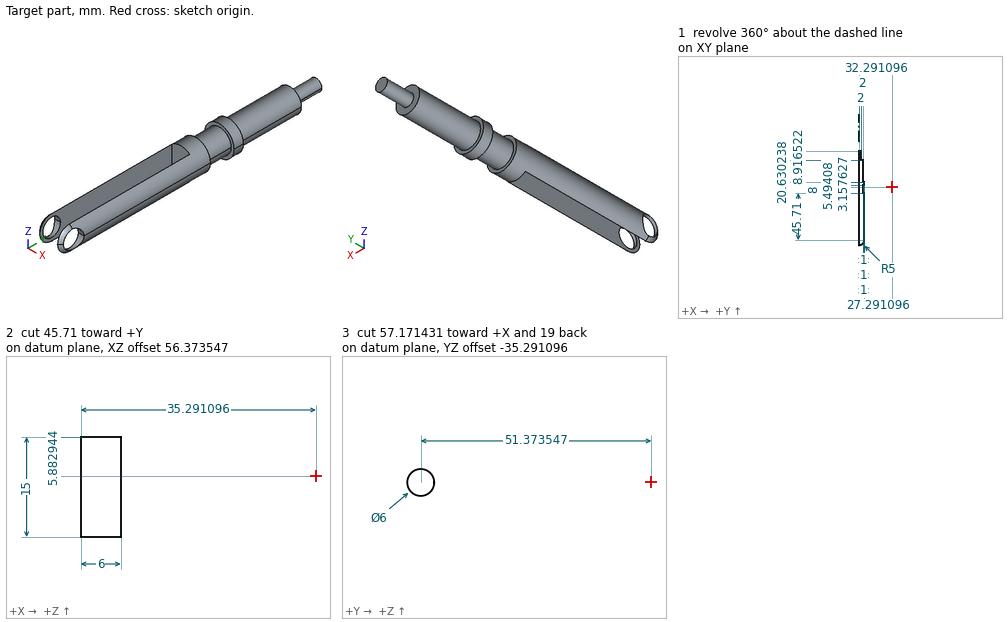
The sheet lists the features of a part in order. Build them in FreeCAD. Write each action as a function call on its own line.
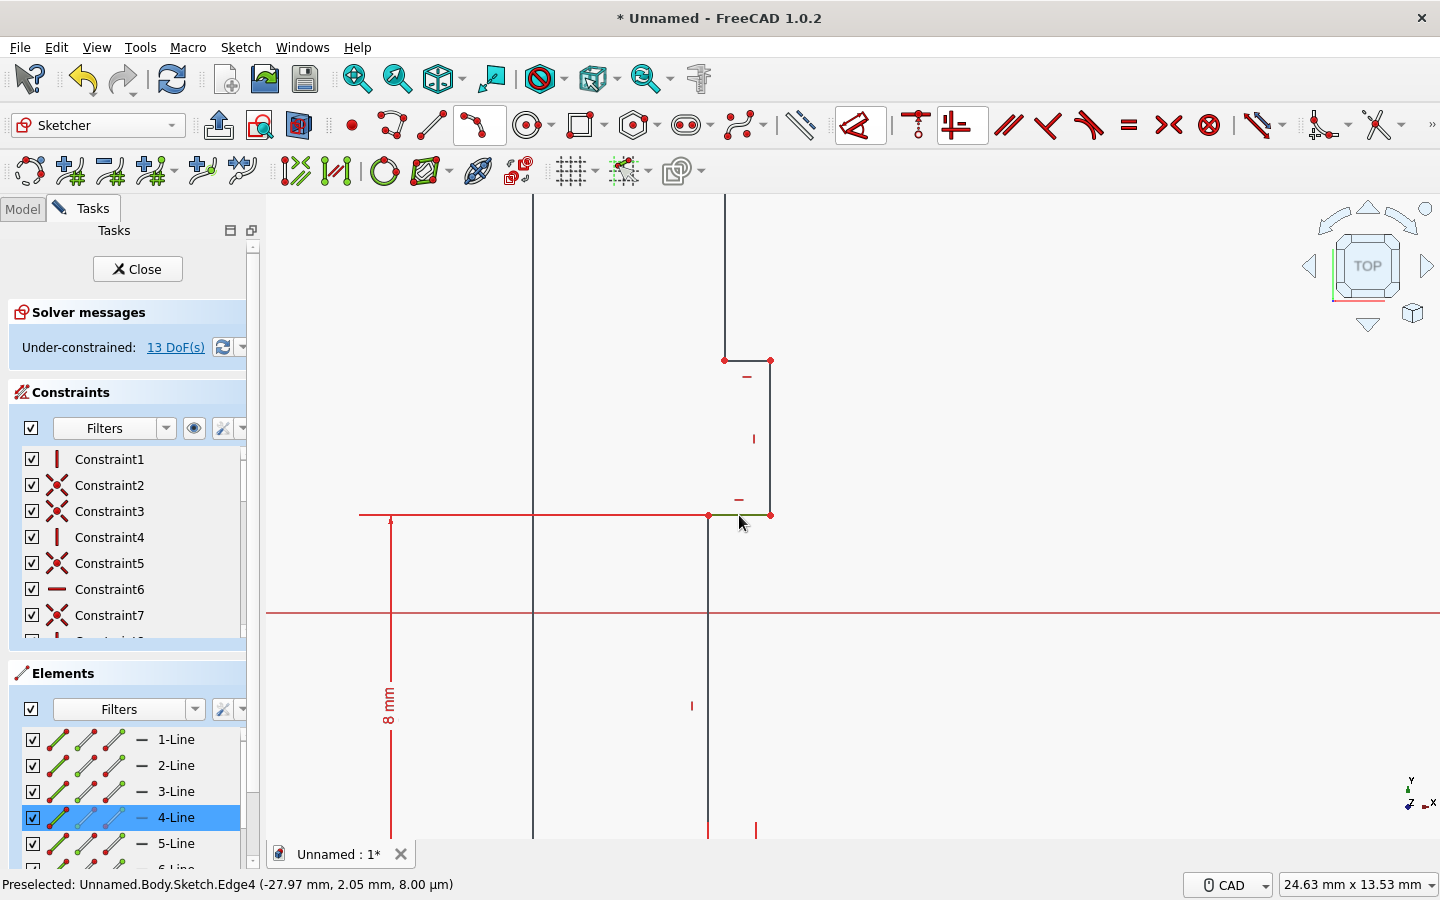
key(l)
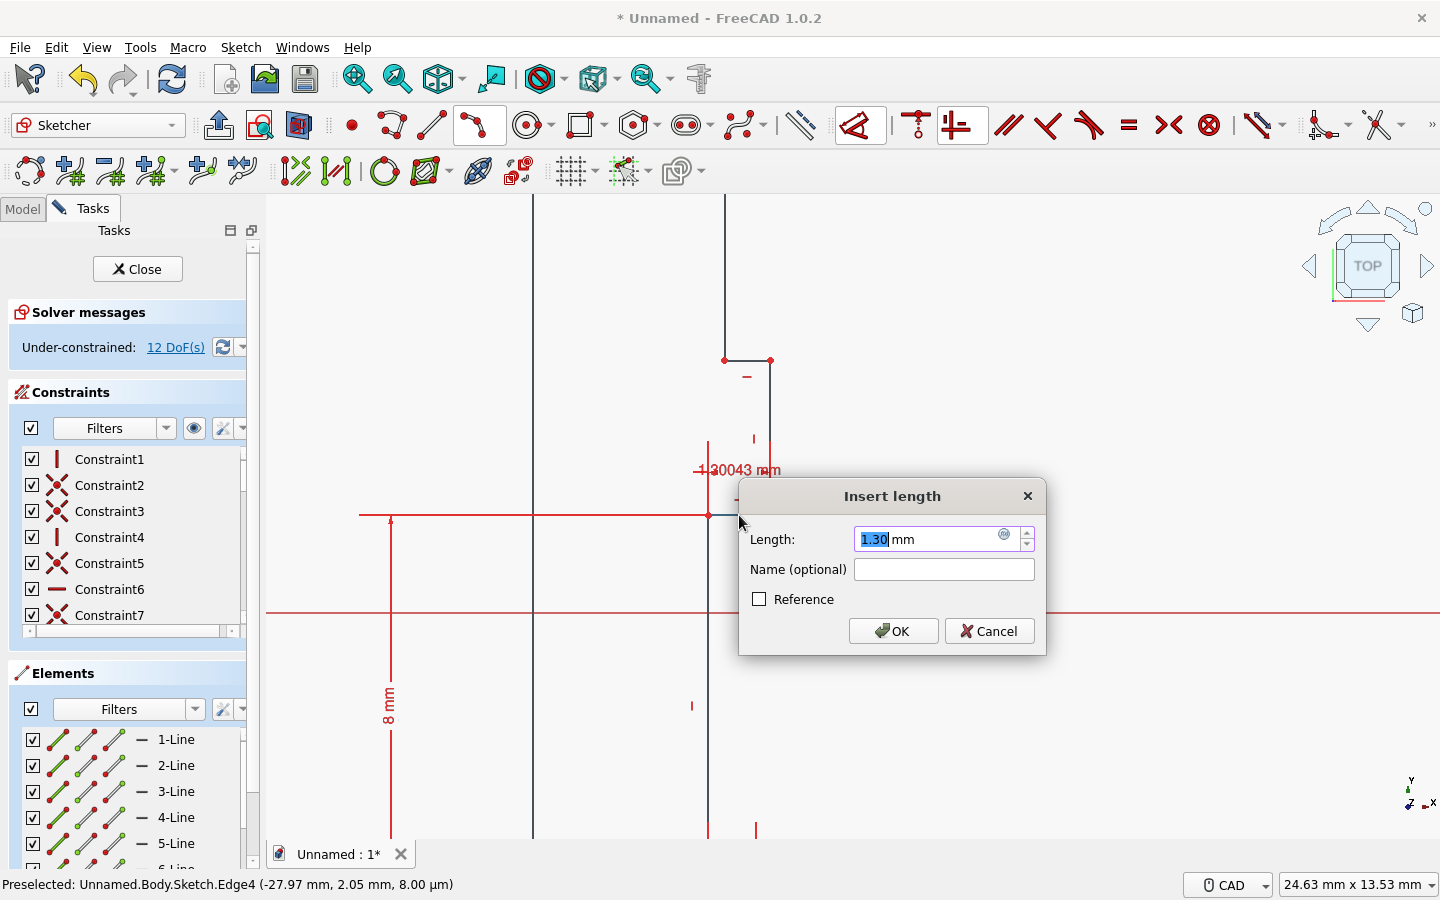
text(1)
key(Return)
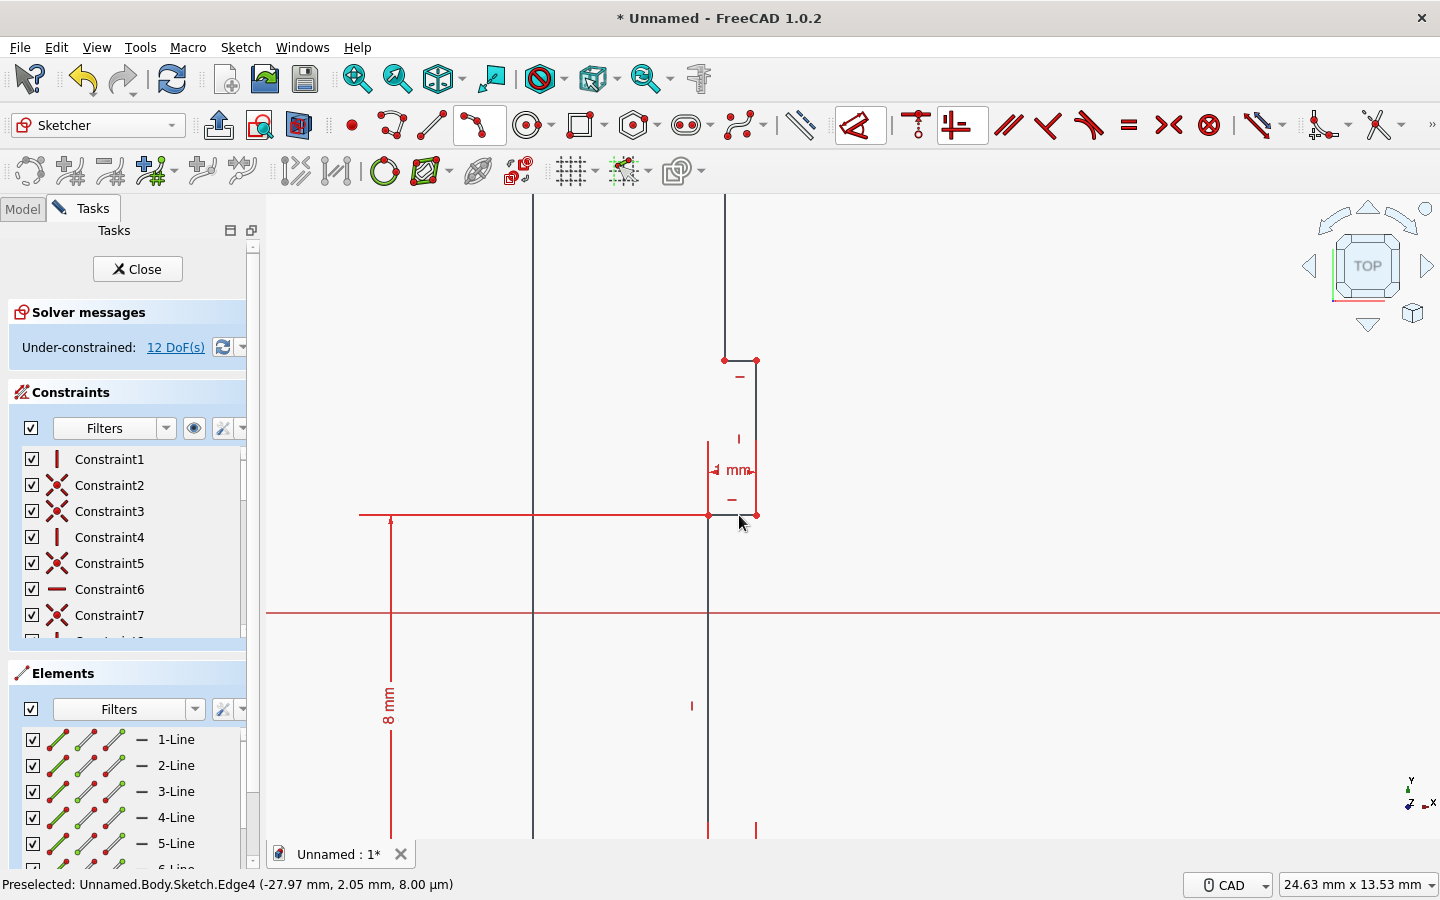
click(747, 361)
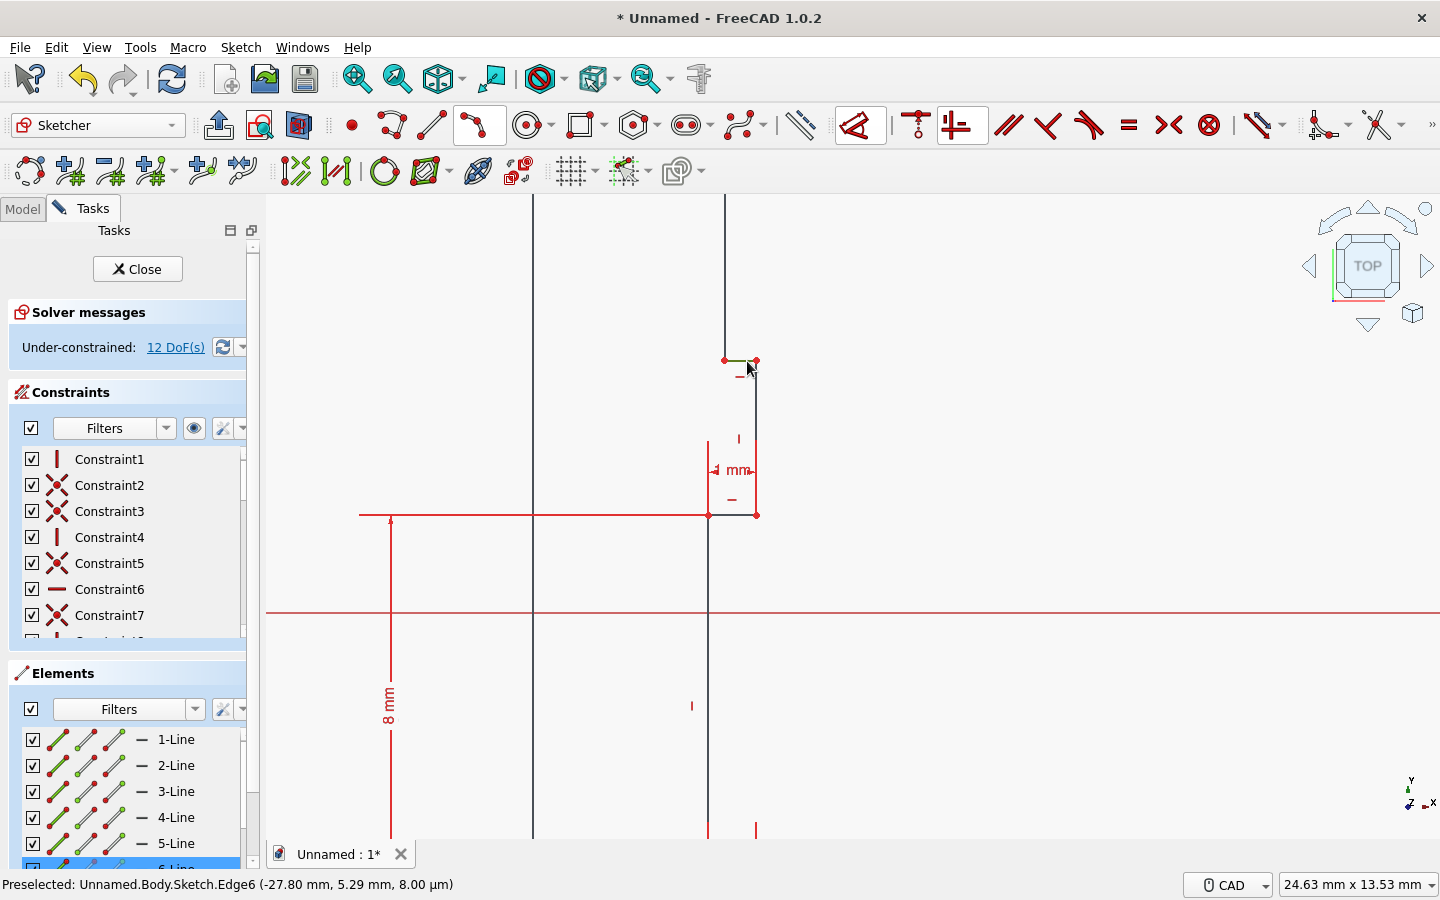
click(880, 126)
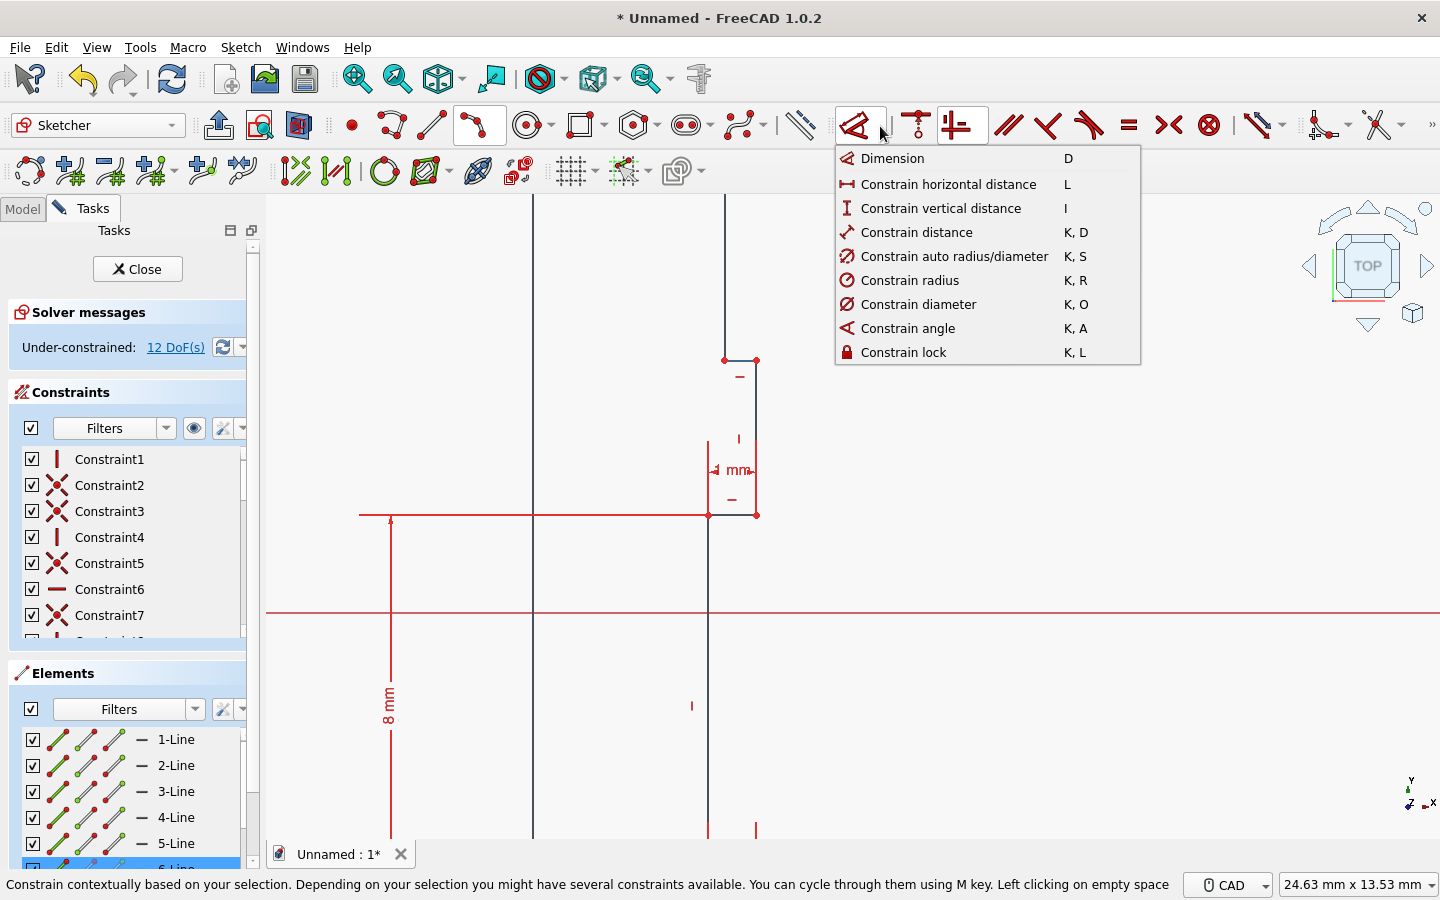
click(988, 184)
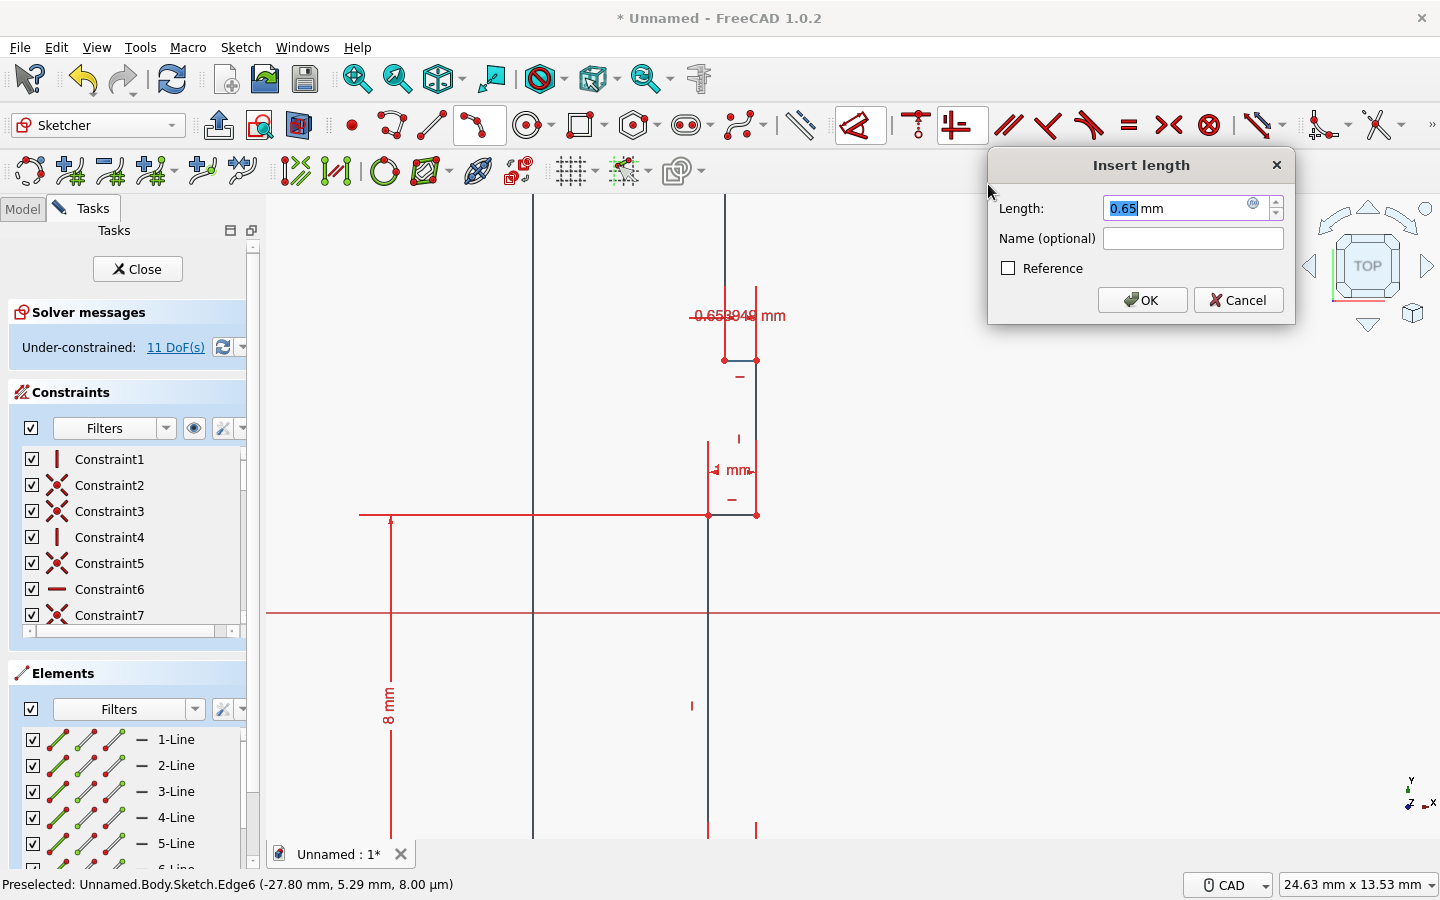
text(1)
key(Return)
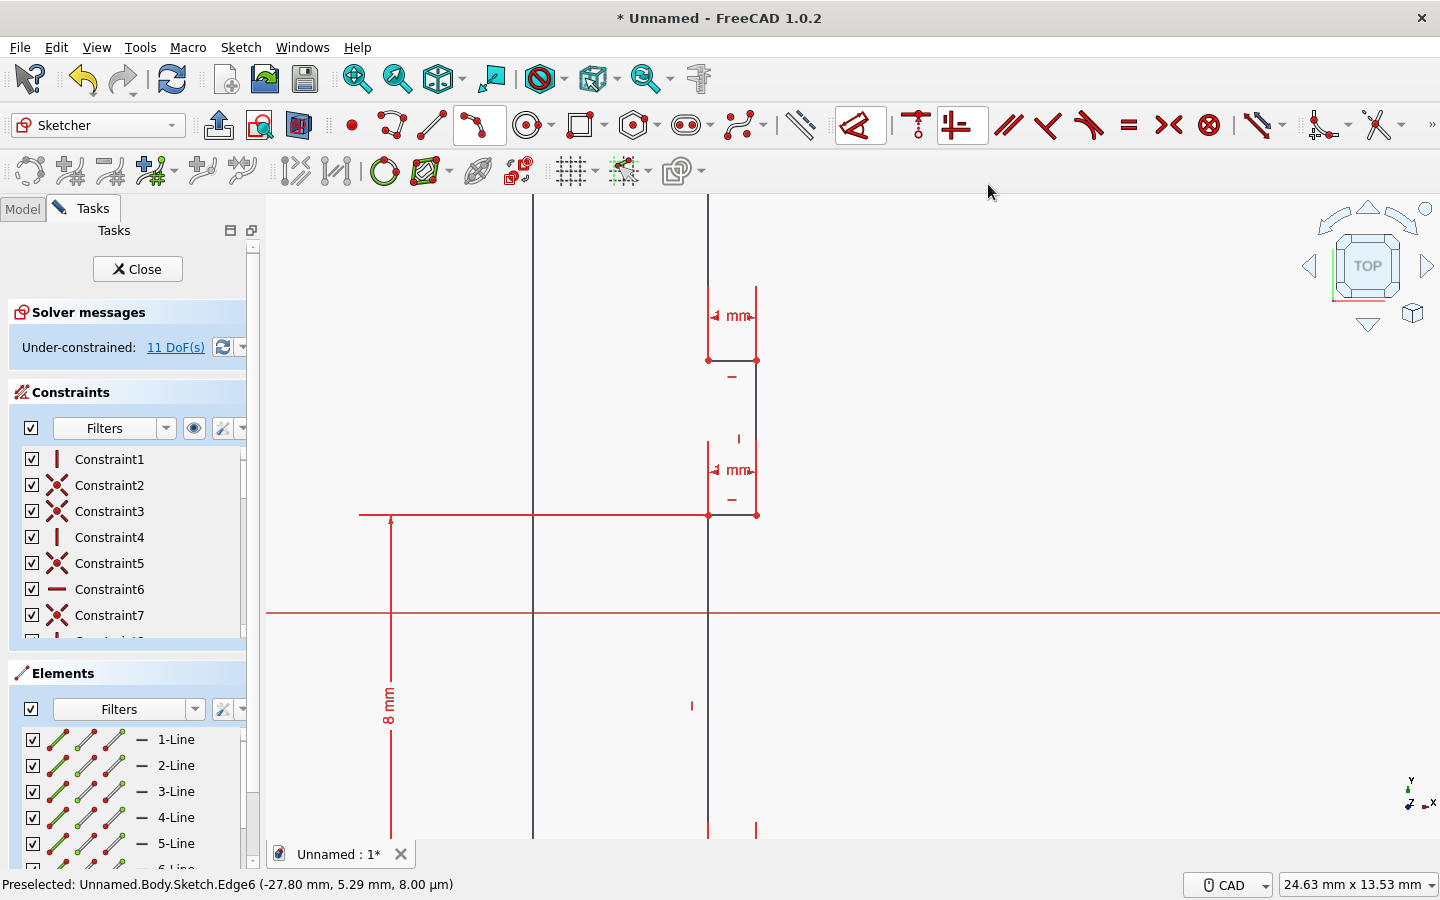
scroll(743, 538, down, 13)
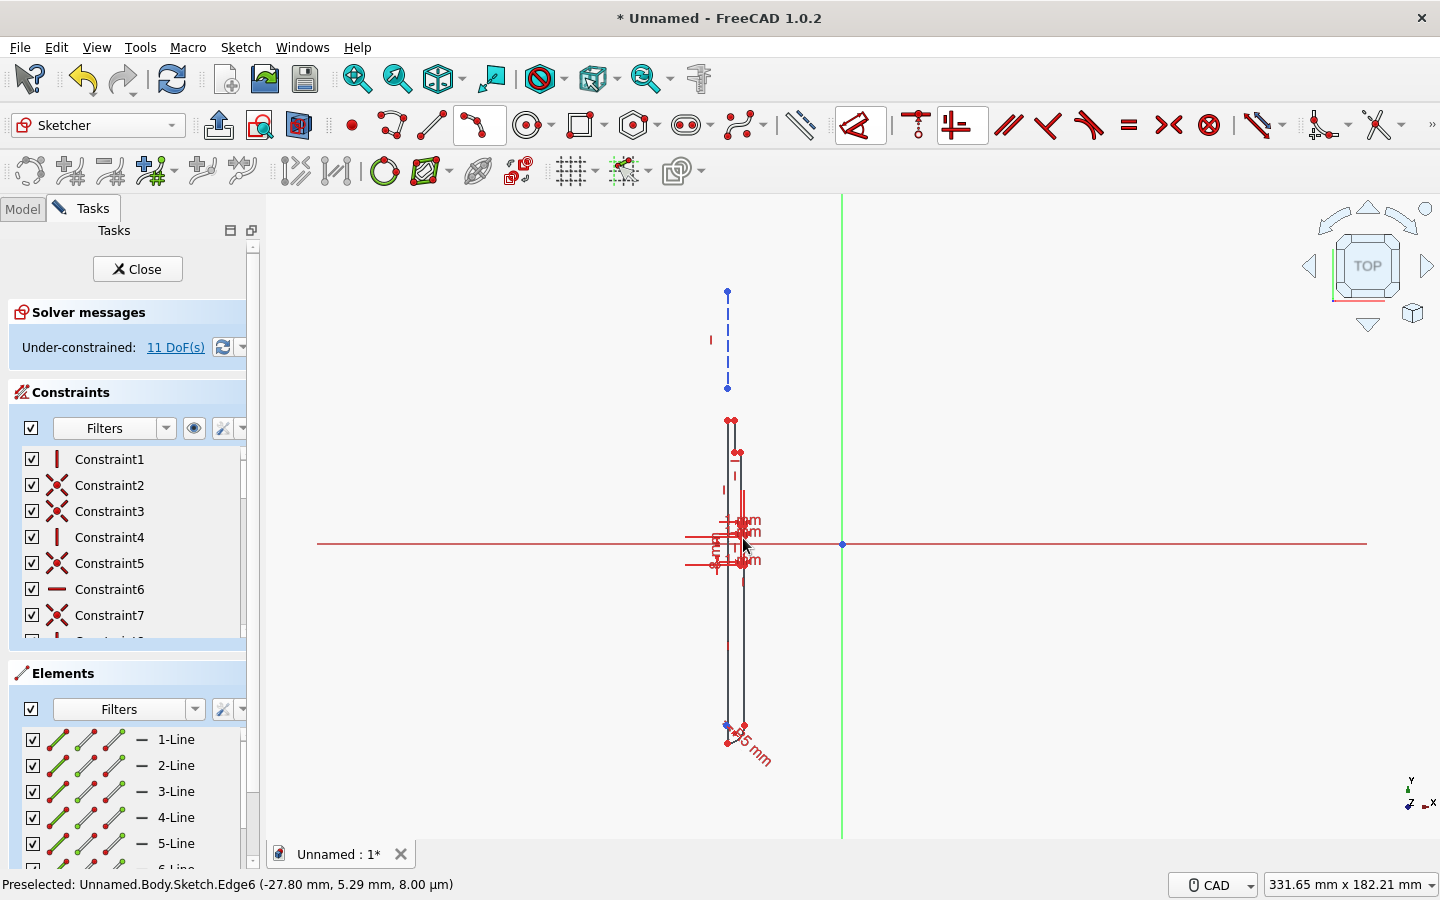
scroll(739, 453, up, 11)